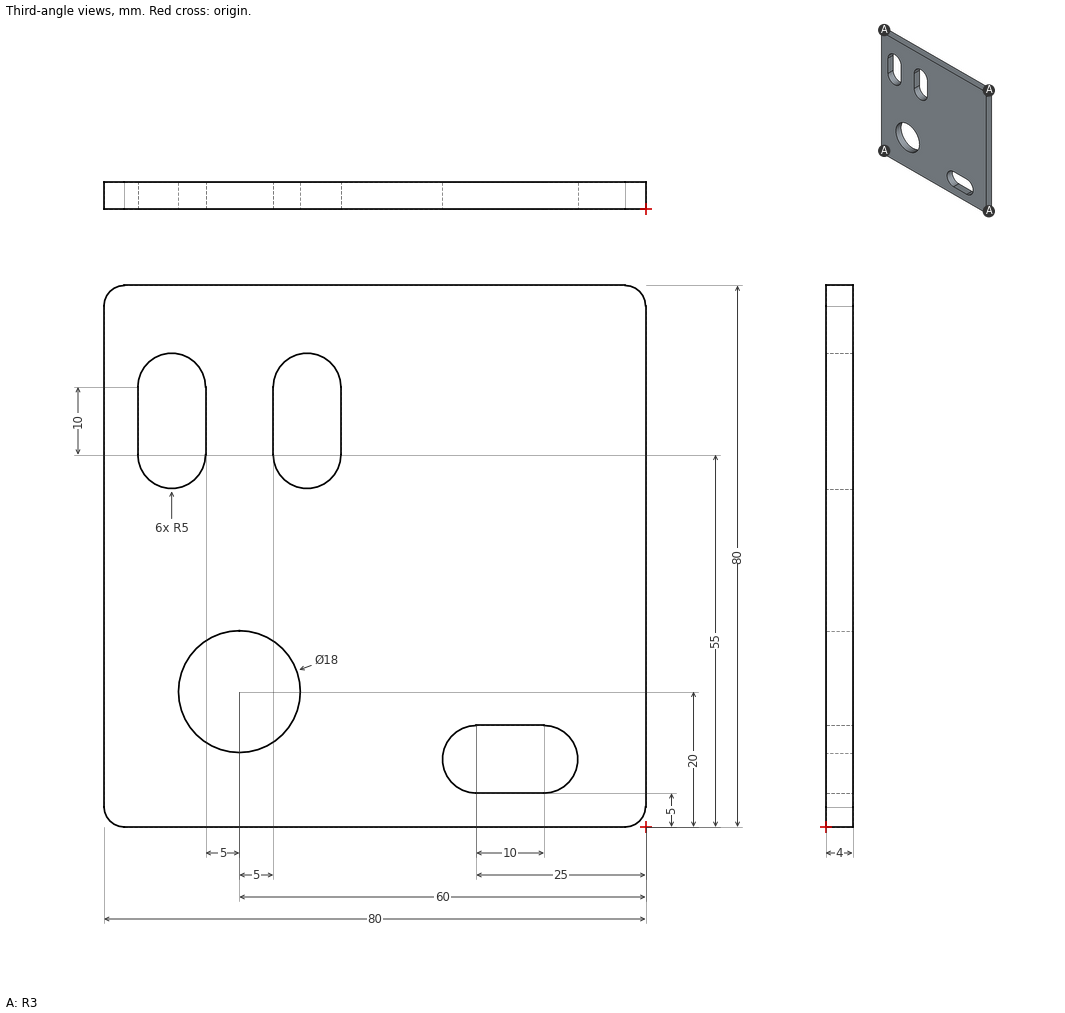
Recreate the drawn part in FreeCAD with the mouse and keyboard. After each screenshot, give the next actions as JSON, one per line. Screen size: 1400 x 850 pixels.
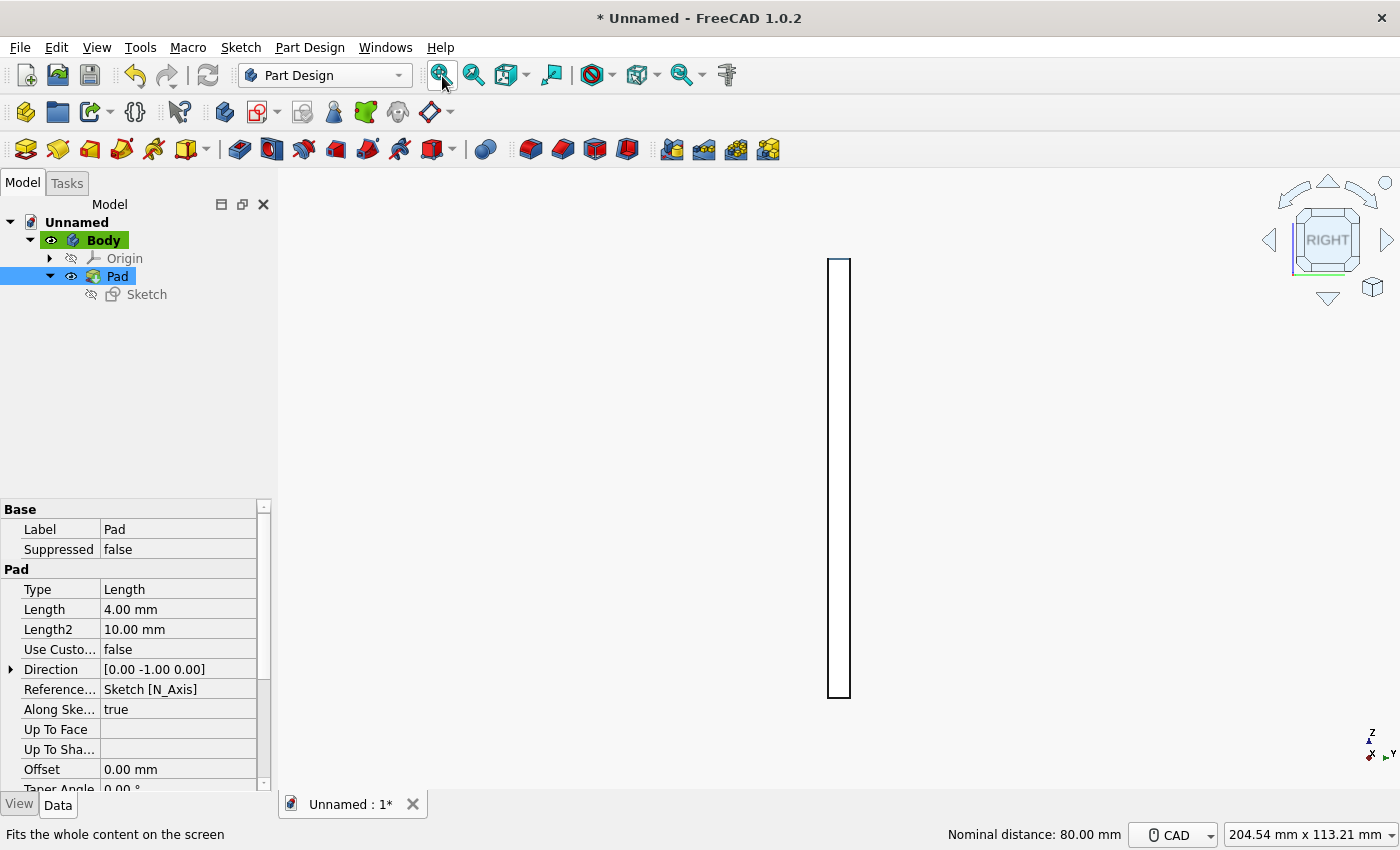
{"action": "left_click", "coordinate": [839, 697], "text": "ctrl"}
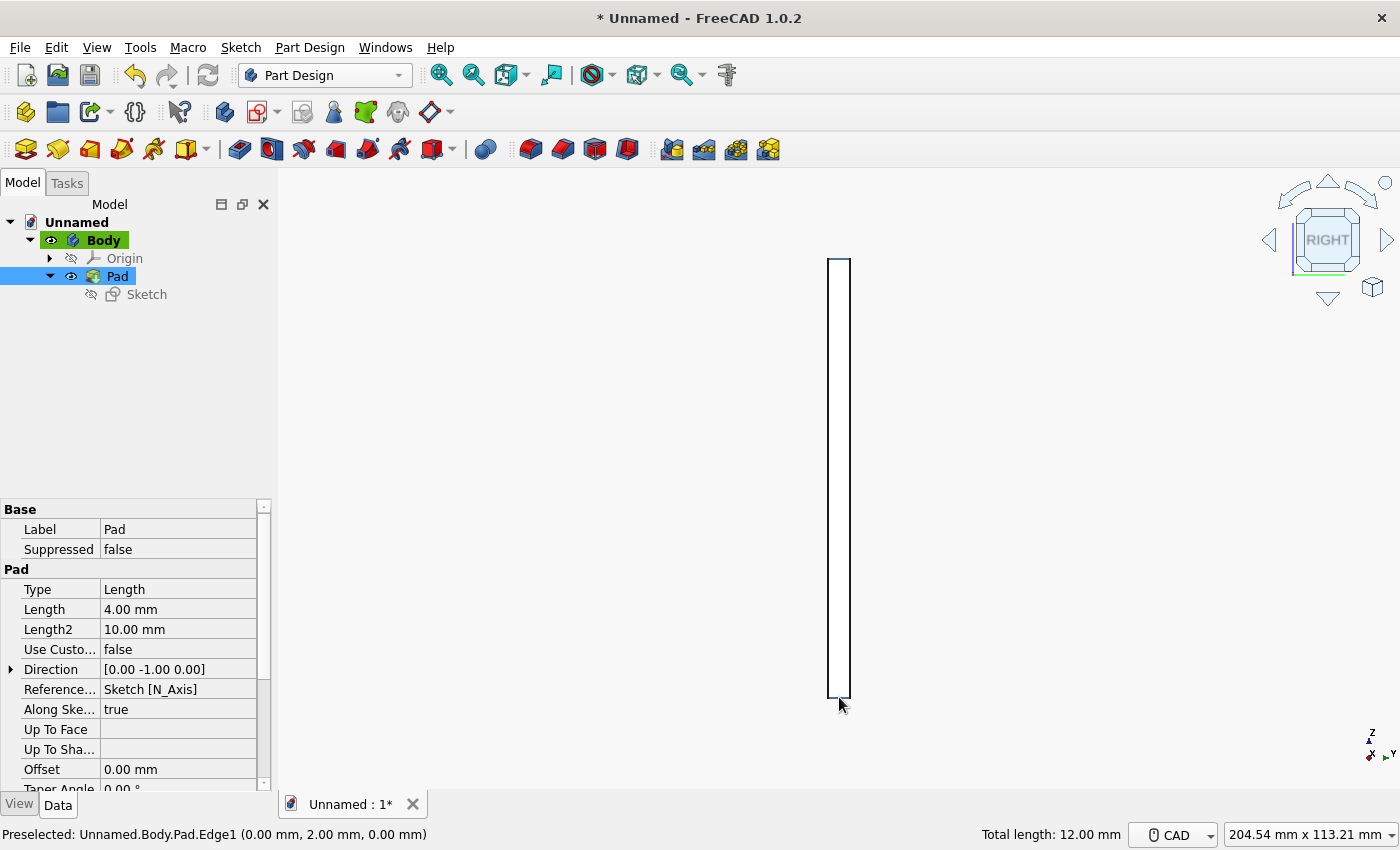
{"action": "scroll", "coordinate": [839, 697], "scroll_direction": "up", "scroll_amount": 4}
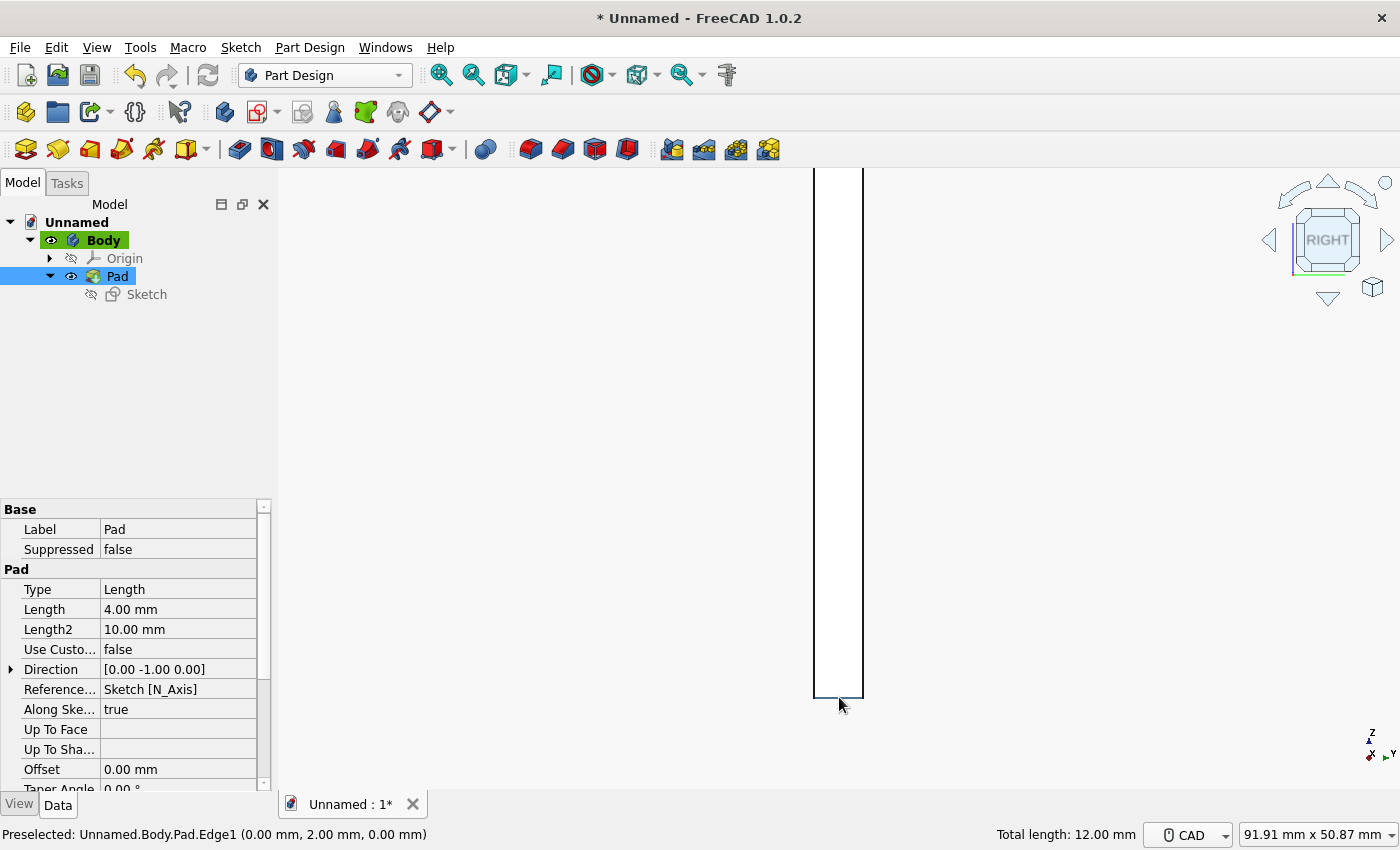
{"action": "left_click", "coordinate": [442, 76]}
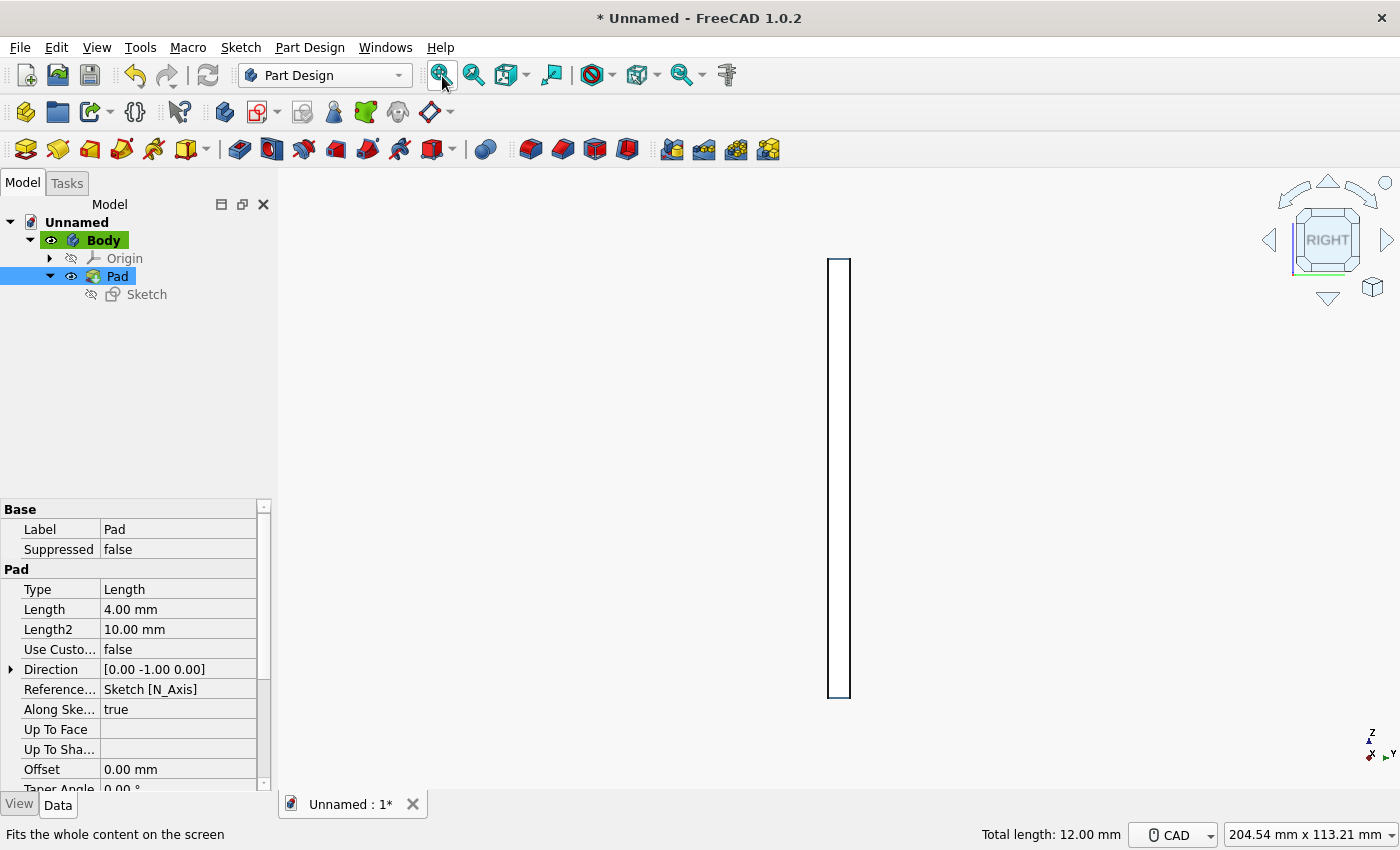
{"action": "key", "text": "5"}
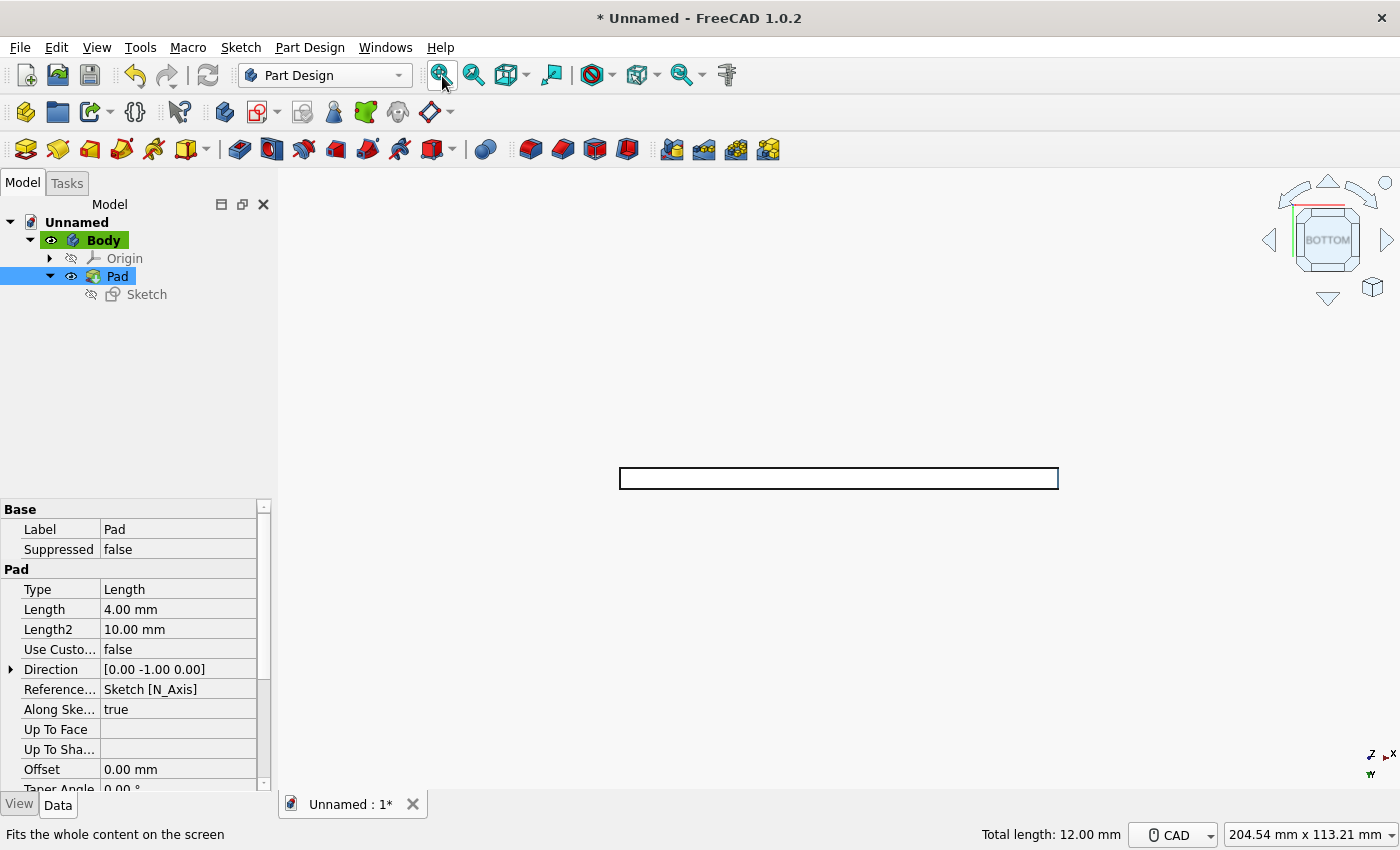
{"action": "left_click", "coordinate": [442, 76]}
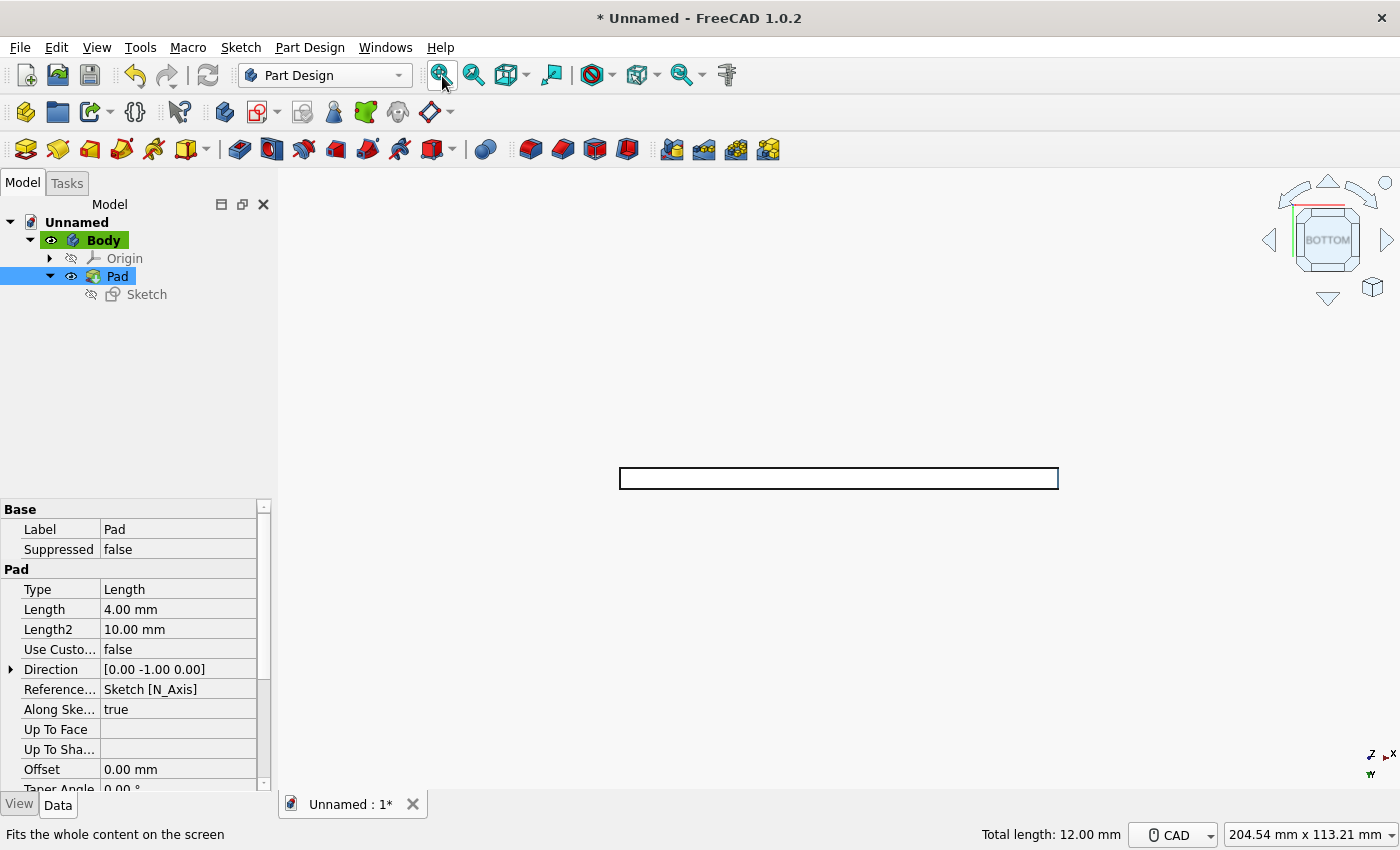
{"action": "left_click", "coordinate": [620, 478], "text": "ctrl"}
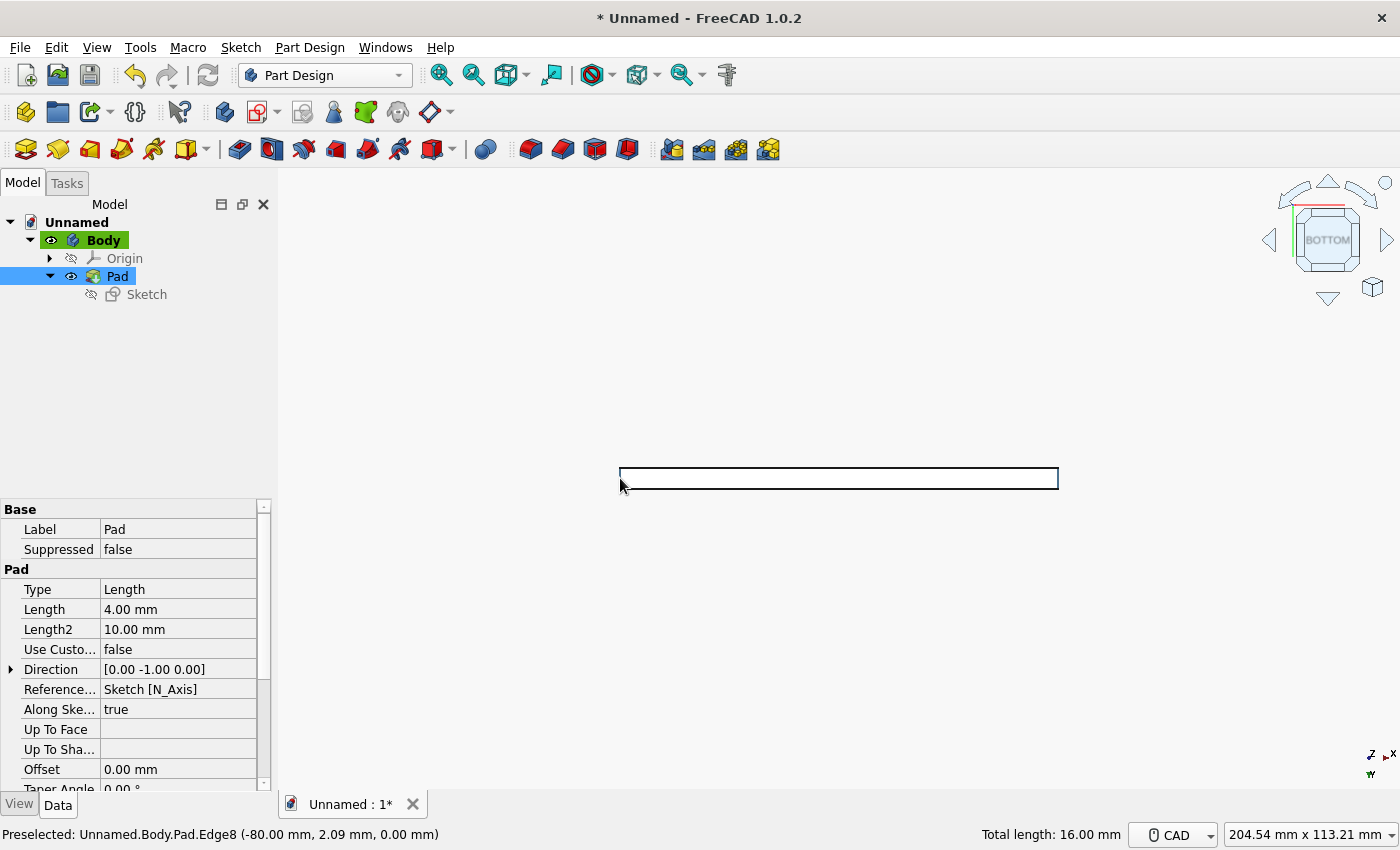
{"action": "left_click", "coordinate": [532, 150]}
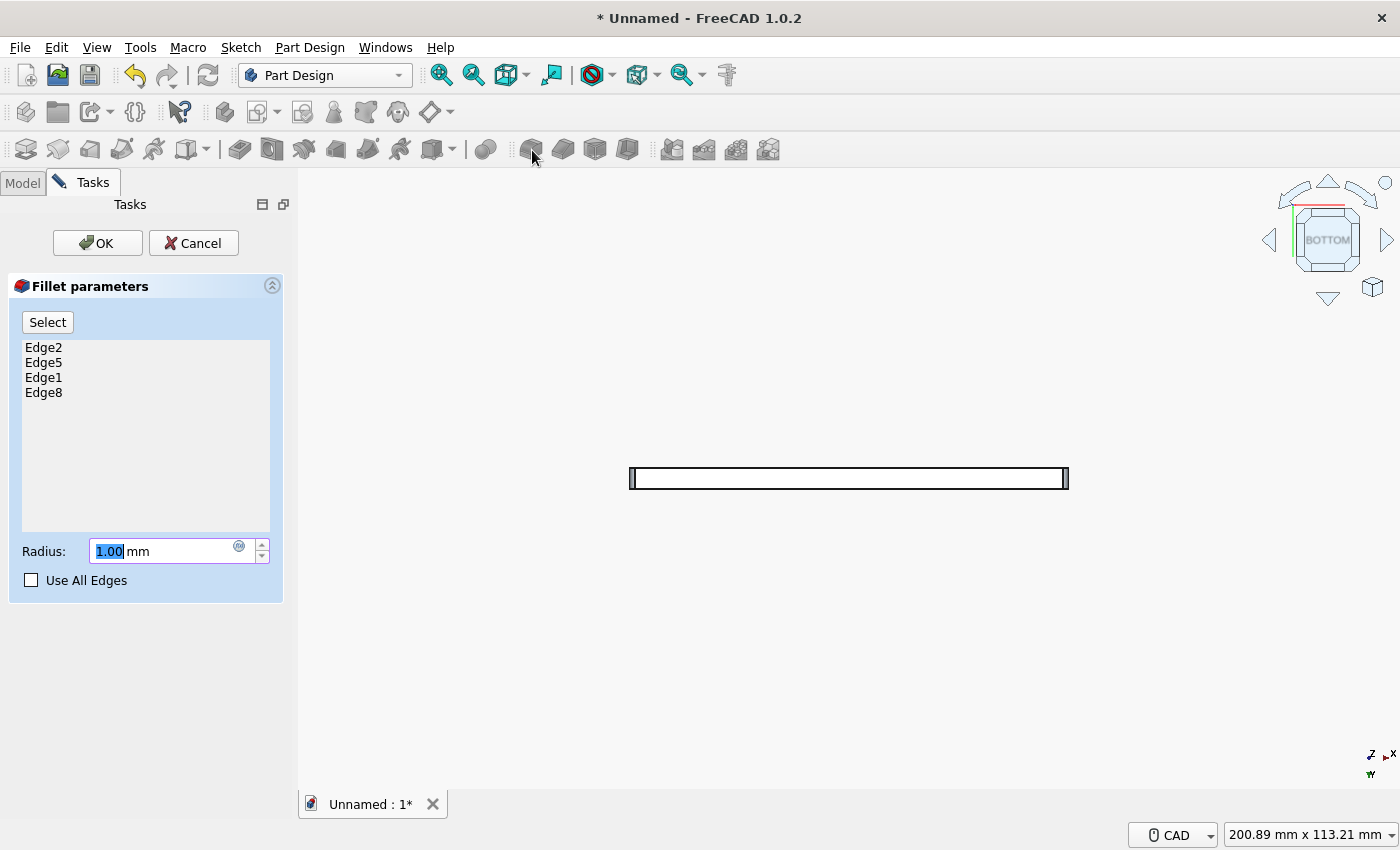
{"action": "type", "text": "3"}
{"action": "key", "text": "Tab"}